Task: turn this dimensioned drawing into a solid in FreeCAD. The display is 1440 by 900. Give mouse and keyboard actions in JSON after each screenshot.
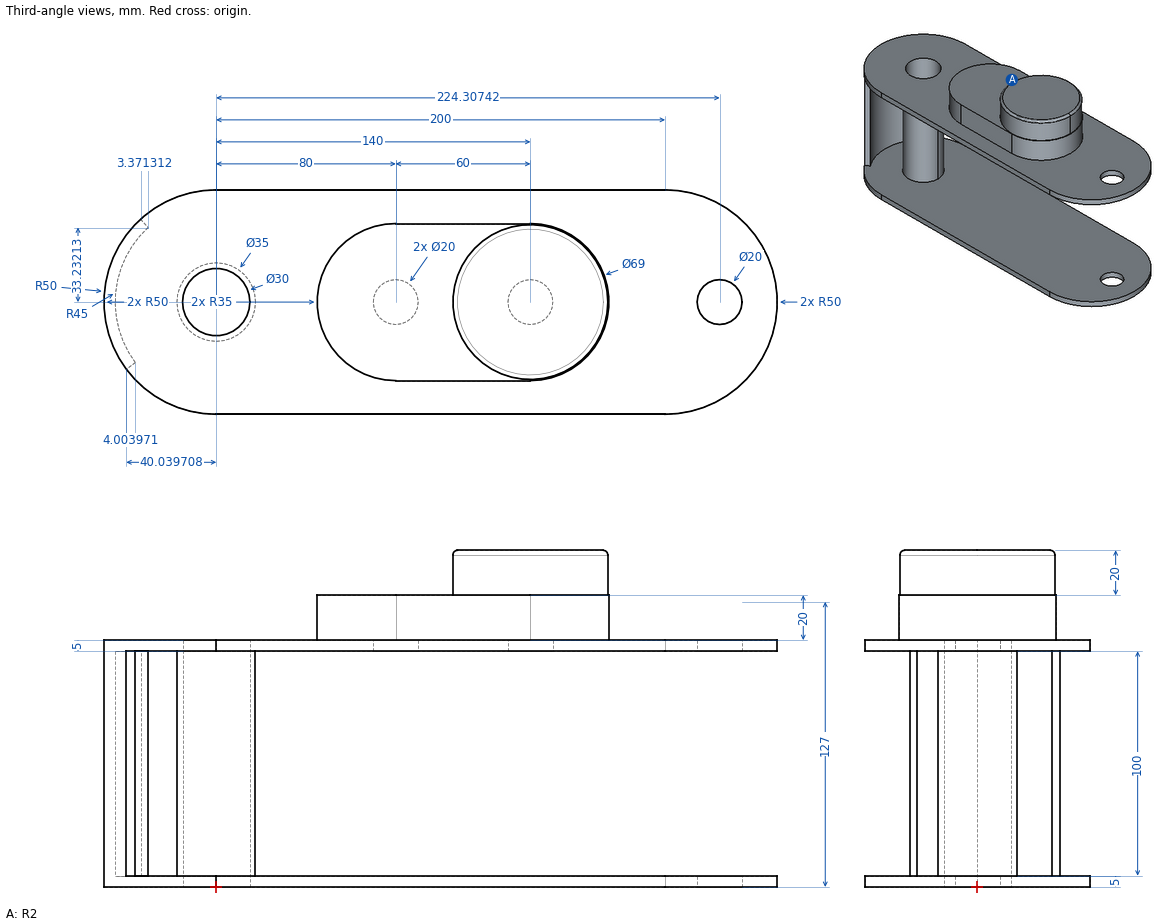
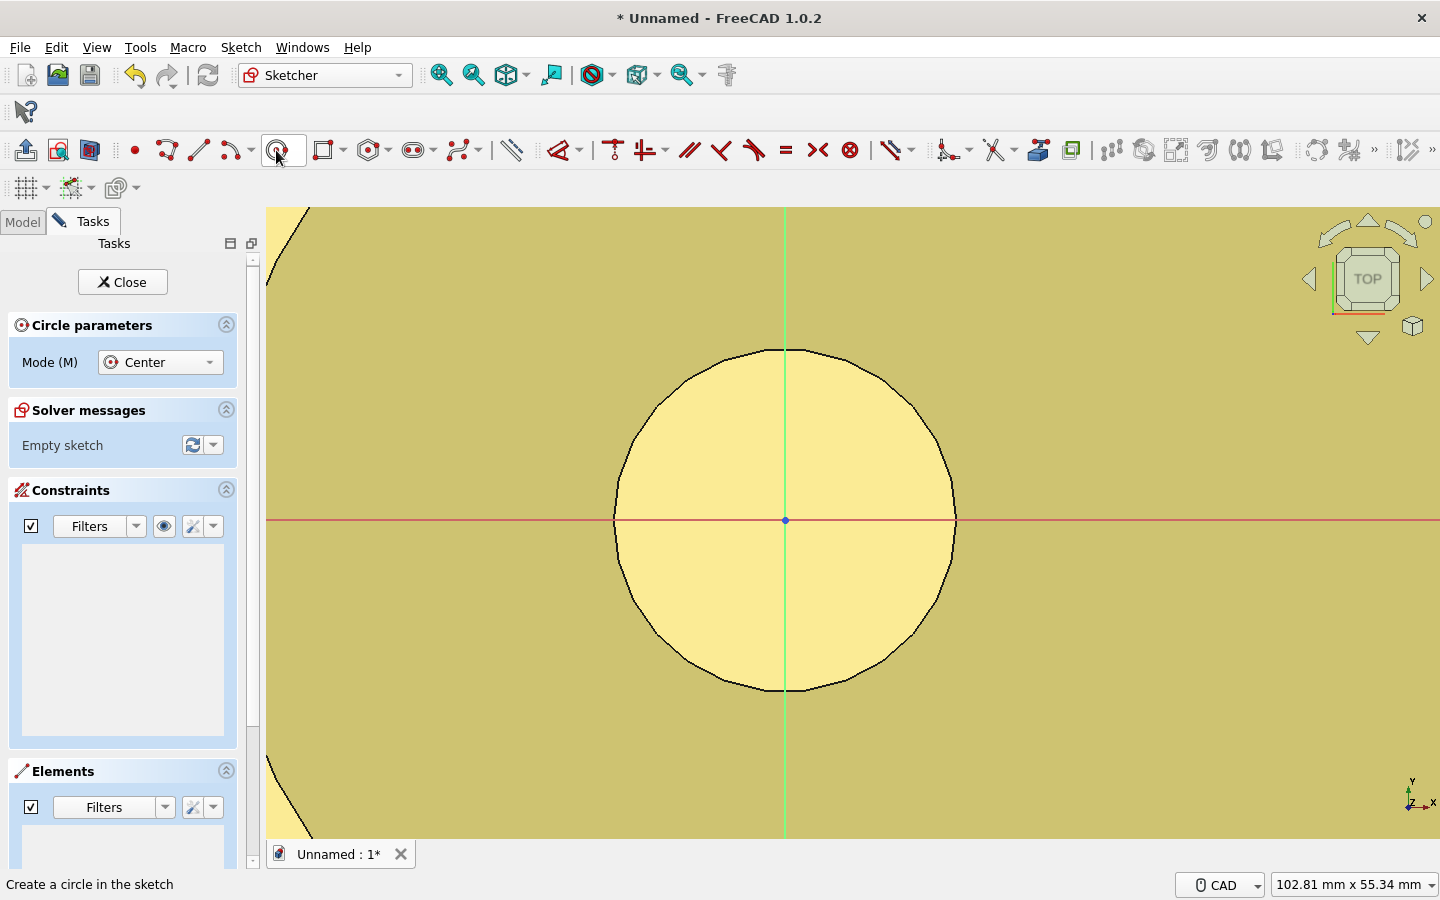
{"action": "left_click", "coordinate": [785, 520]}
{"action": "left_click", "coordinate": [926, 379]}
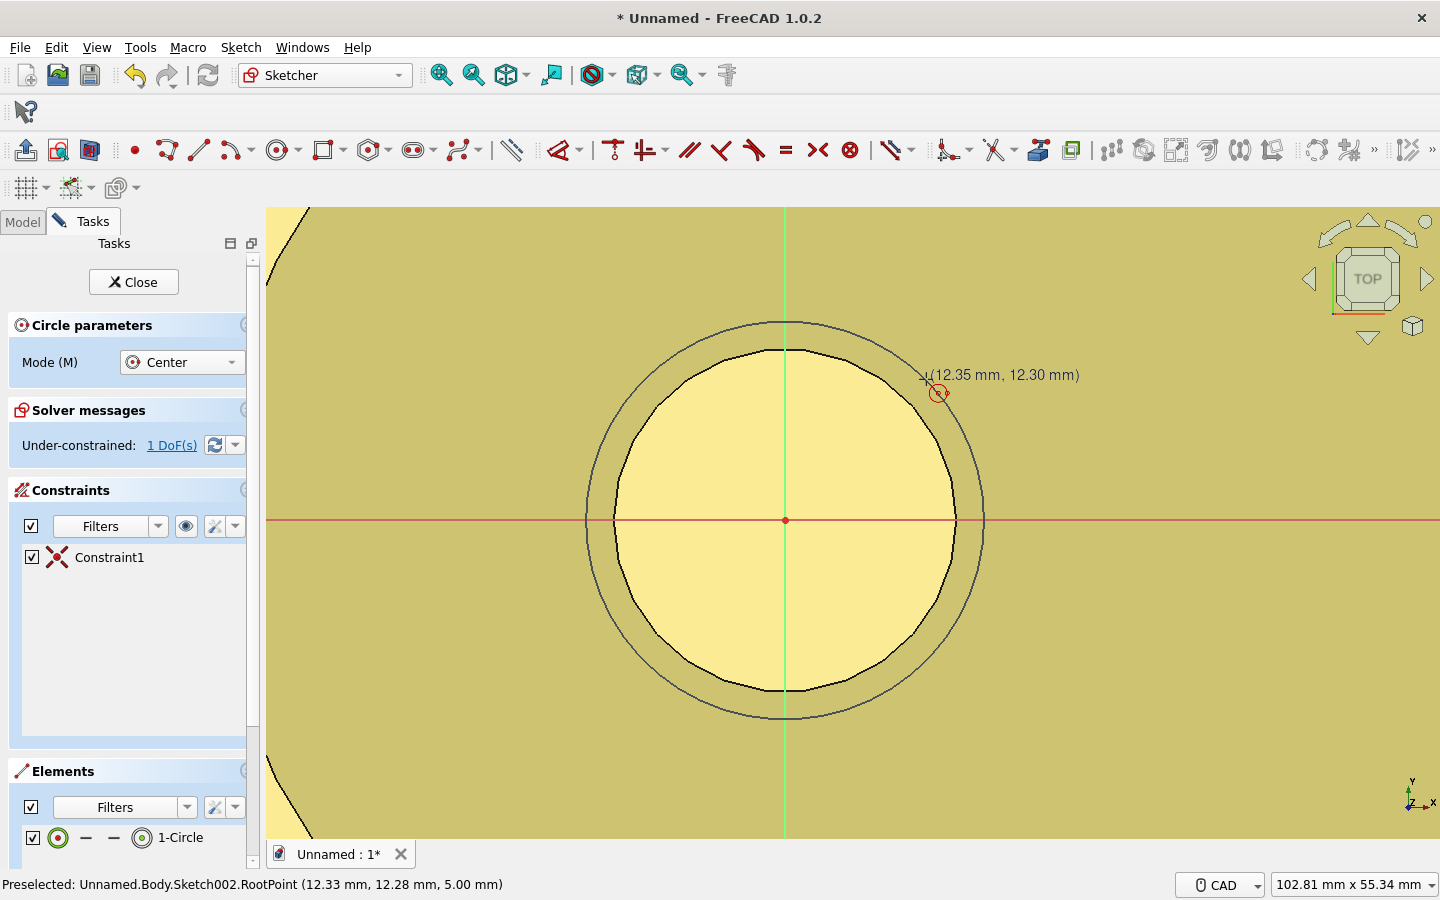
{"action": "left_click", "coordinate": [785, 520]}
{"action": "left_click", "coordinate": [906, 399]}
{"action": "key", "text": "Escape"}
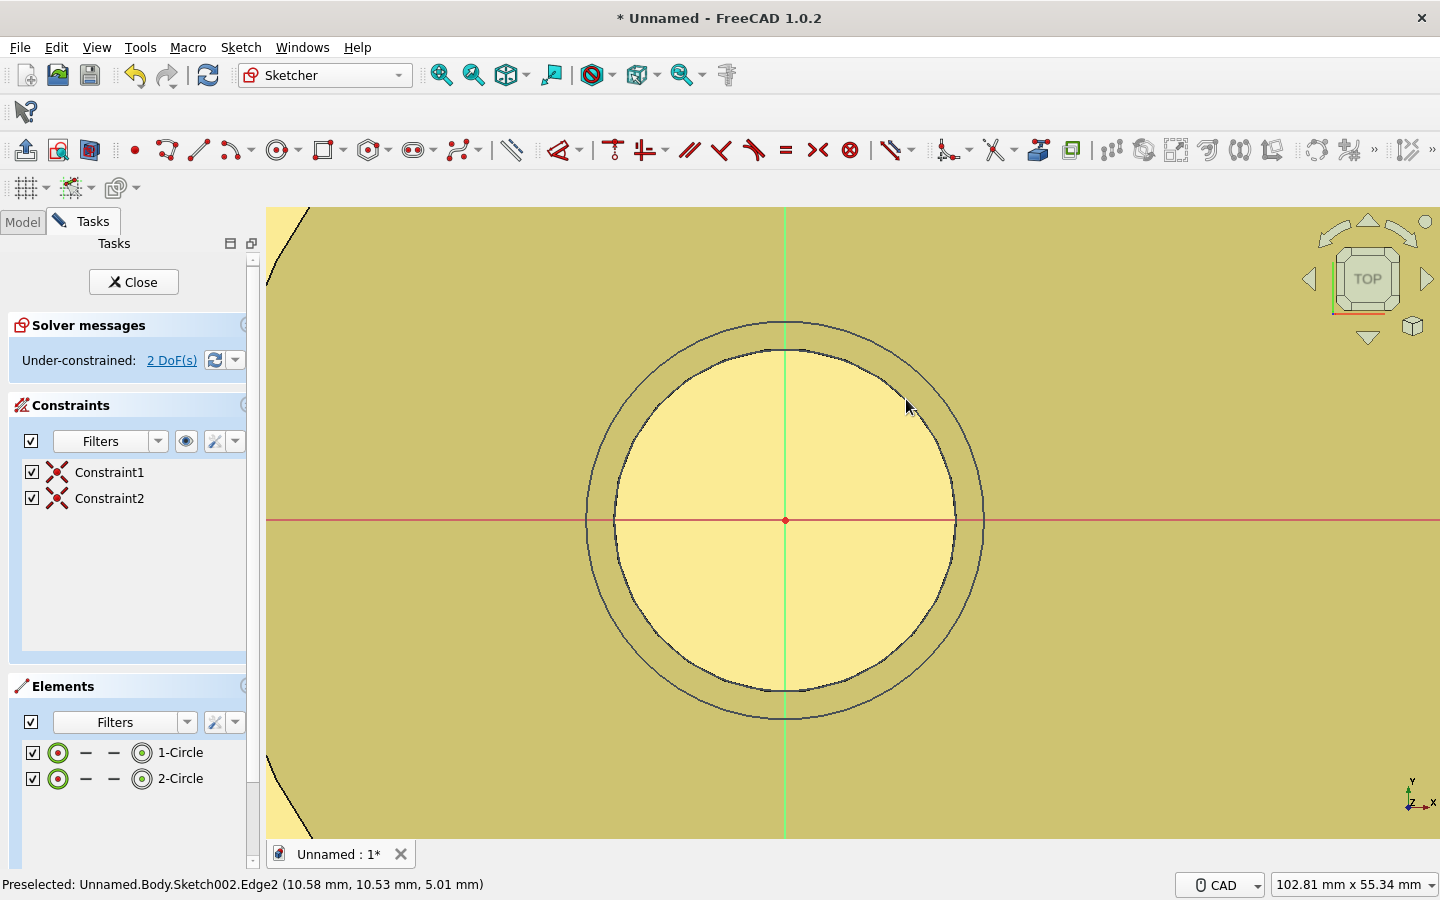
{"action": "left_click", "coordinate": [558, 150]}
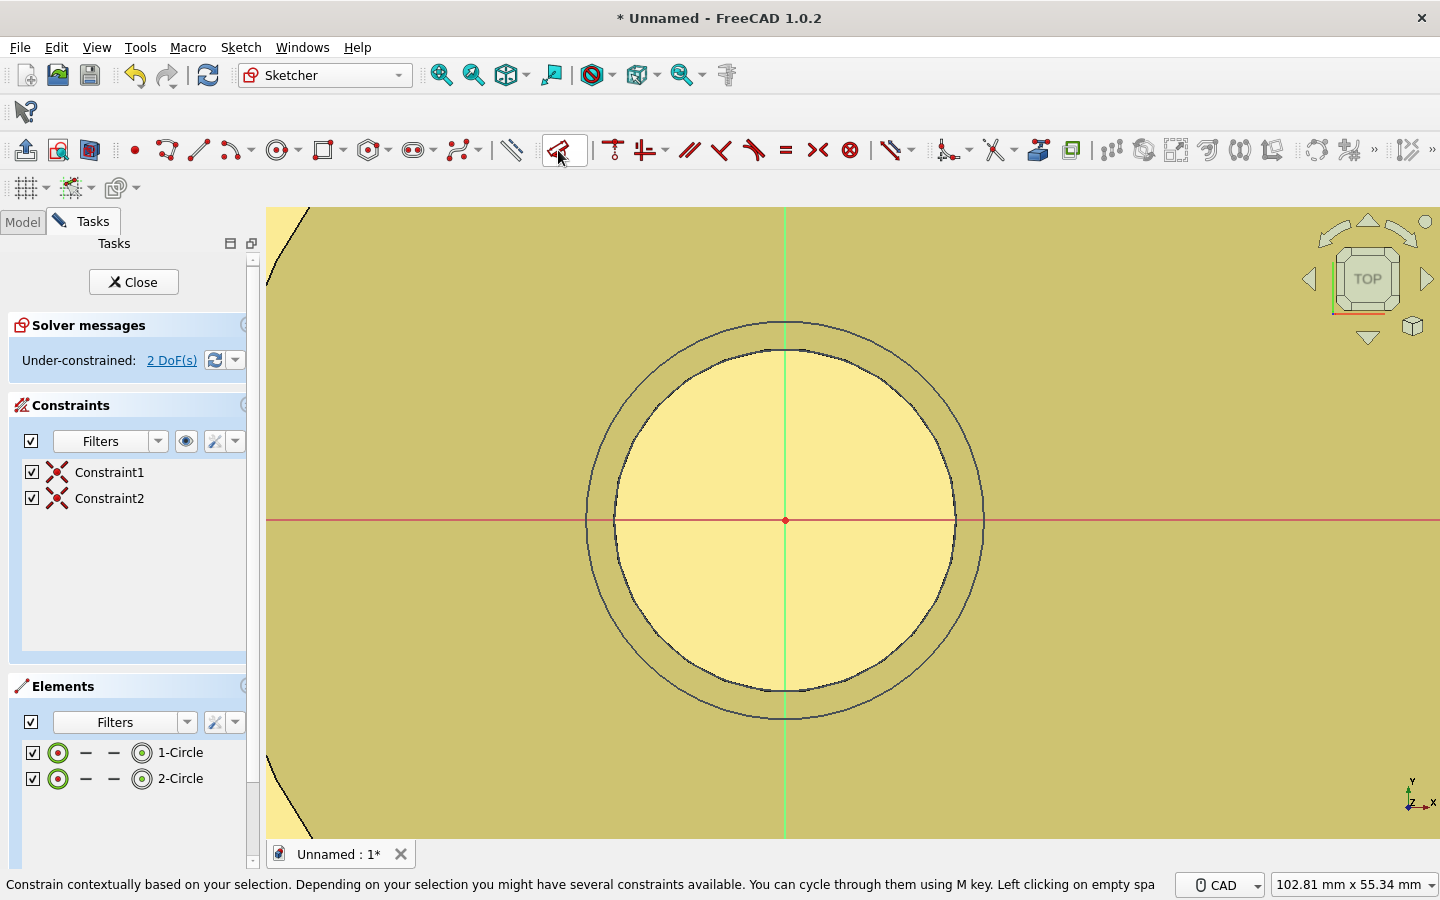
{"action": "left_click", "coordinate": [925, 379]}
{"action": "left_click", "coordinate": [948, 356]}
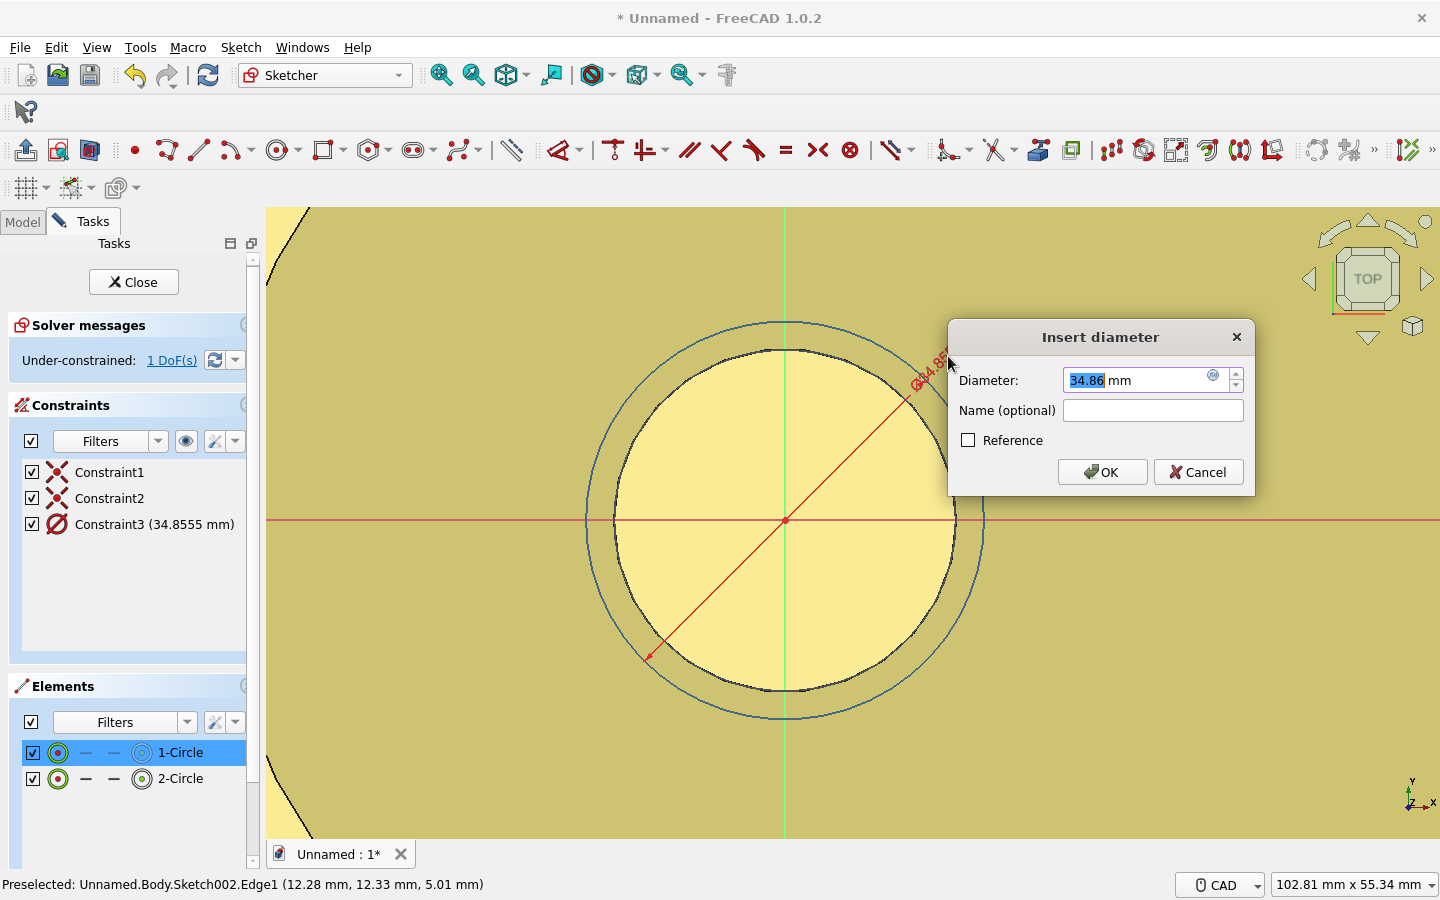
{"action": "type", "text": "35"}
{"action": "key", "text": "Return"}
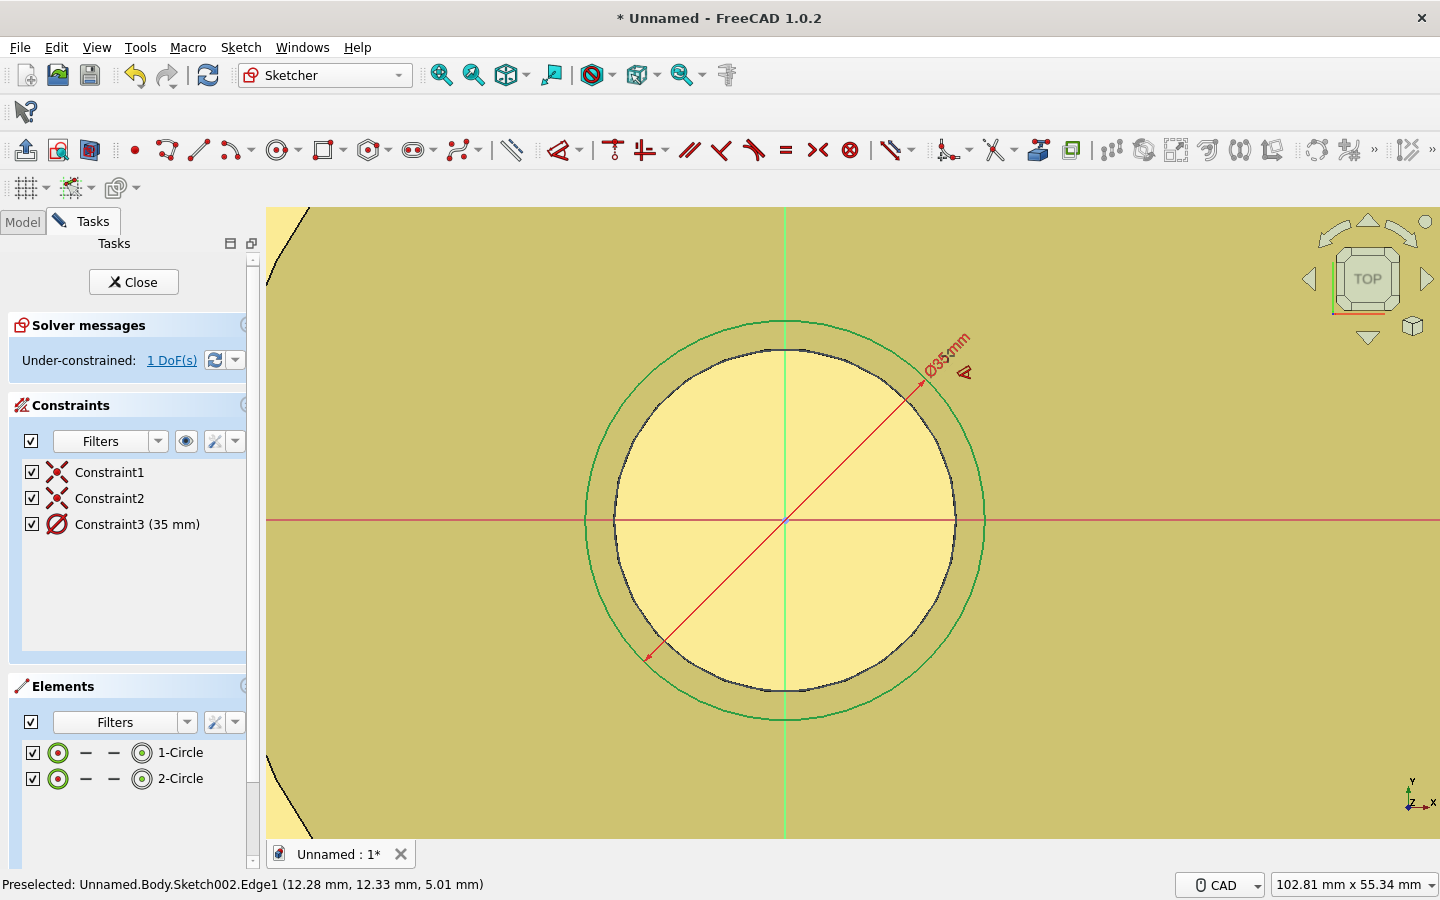
{"action": "left_click", "coordinate": [905, 399]}
{"action": "left_click", "coordinate": [1001, 456]}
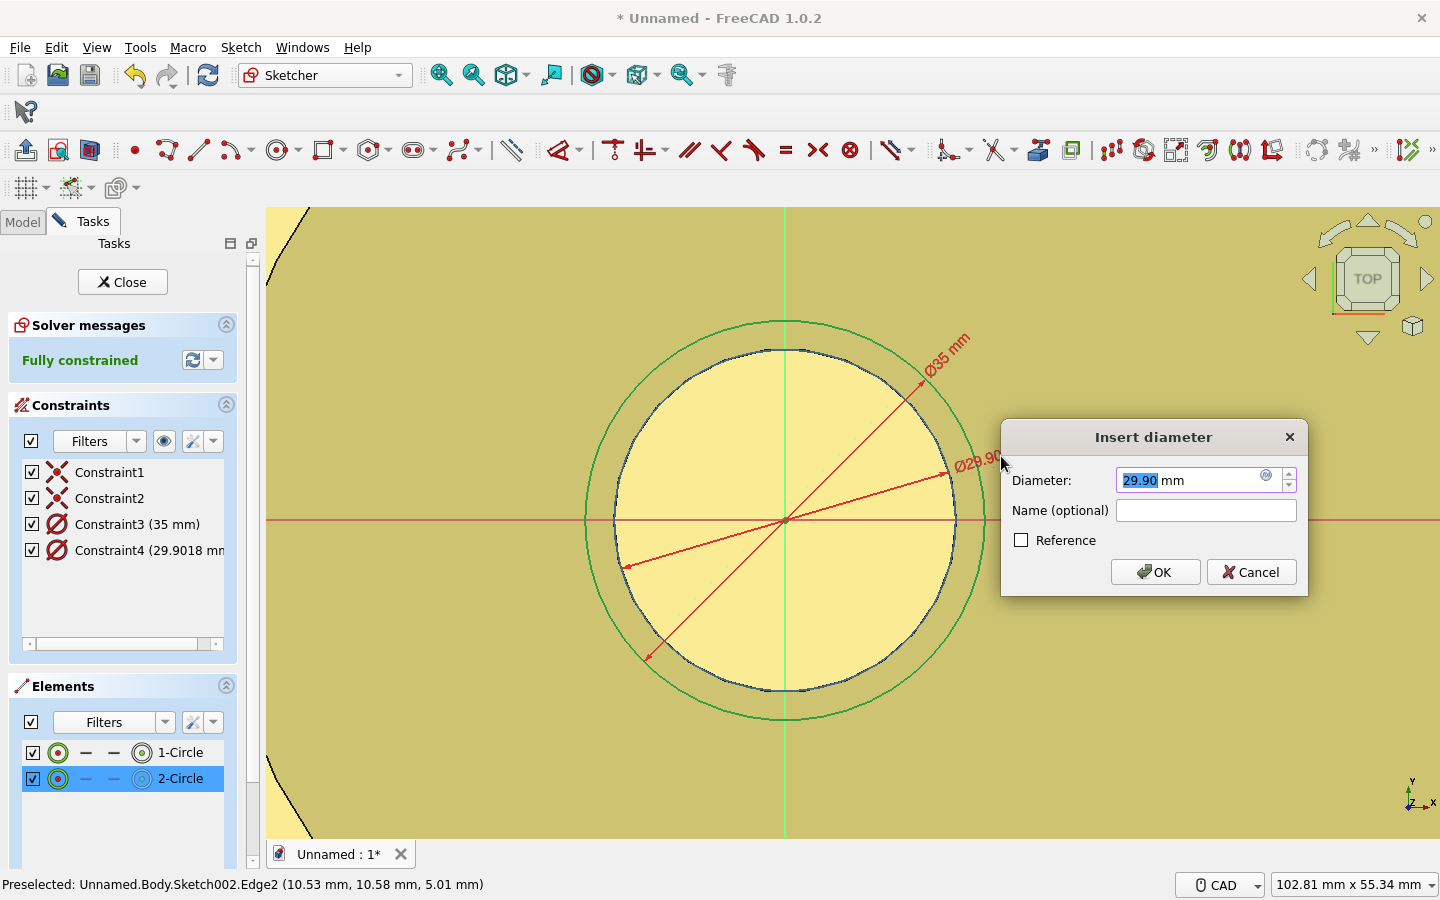
{"action": "type", "text": "30"}
{"action": "key", "text": "Return"}
{"action": "key", "text": "Escape"}